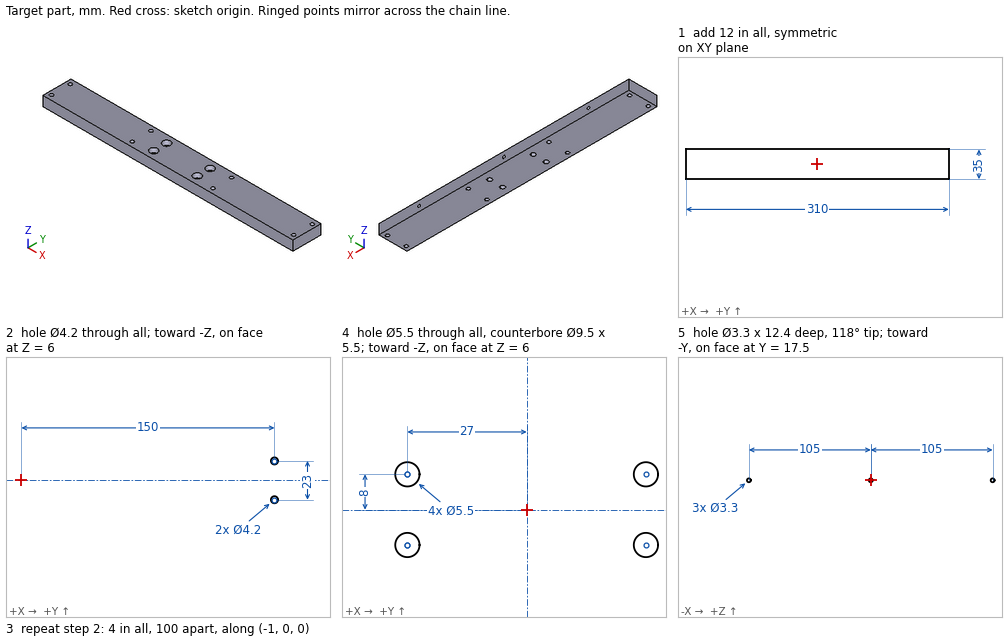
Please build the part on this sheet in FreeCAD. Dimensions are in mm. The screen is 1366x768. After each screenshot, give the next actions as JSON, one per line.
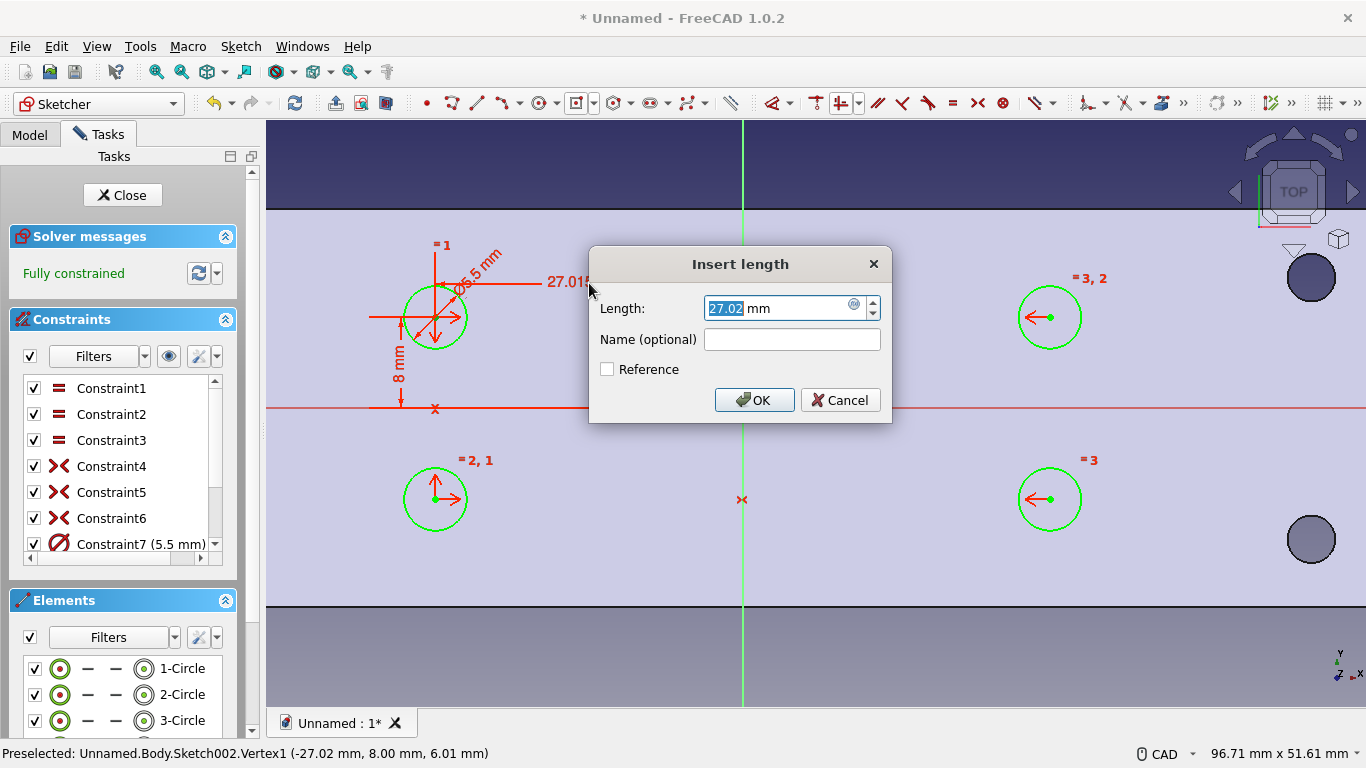
{"action": "type", "text": "27"}
{"action": "key", "text": "Return"}
{"action": "key", "text": "Escape"}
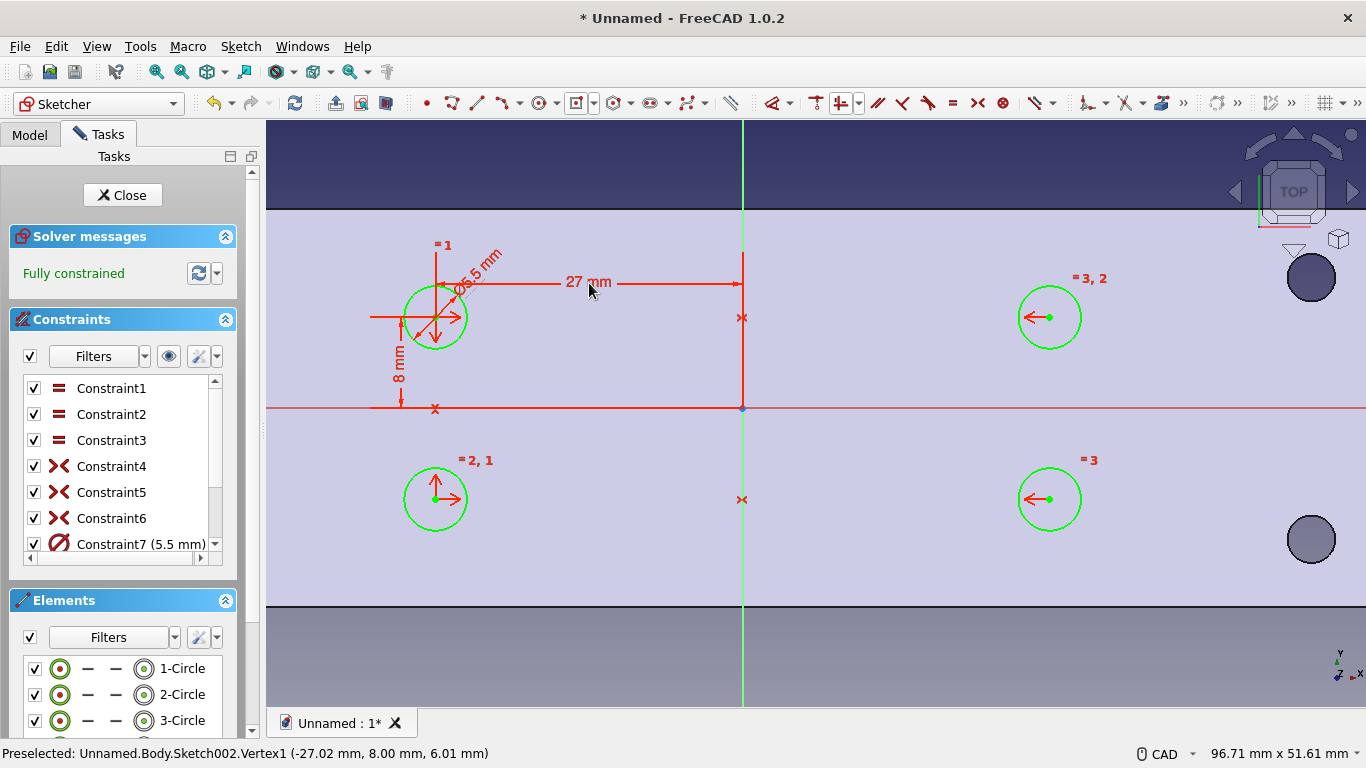
{"action": "left_click", "coordinate": [123, 195]}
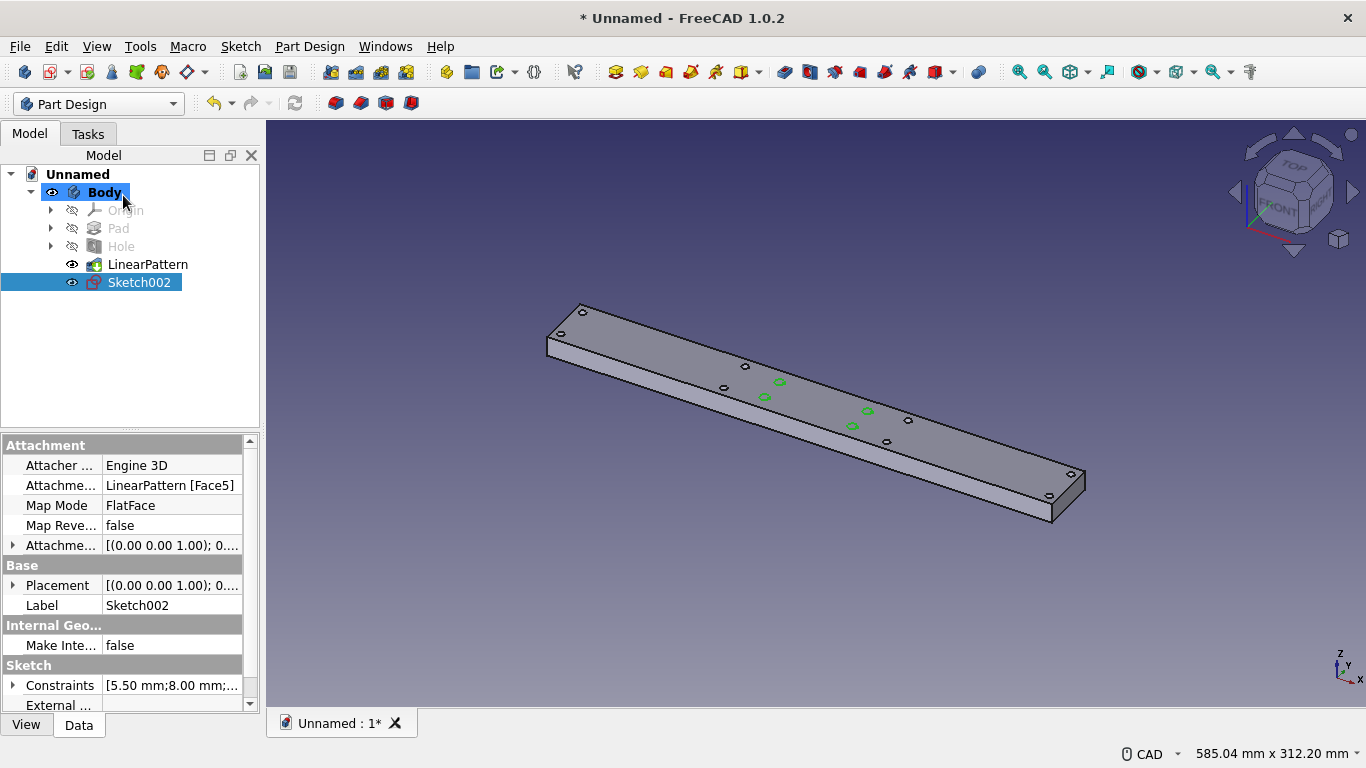
{"action": "left_click", "coordinate": [810, 72]}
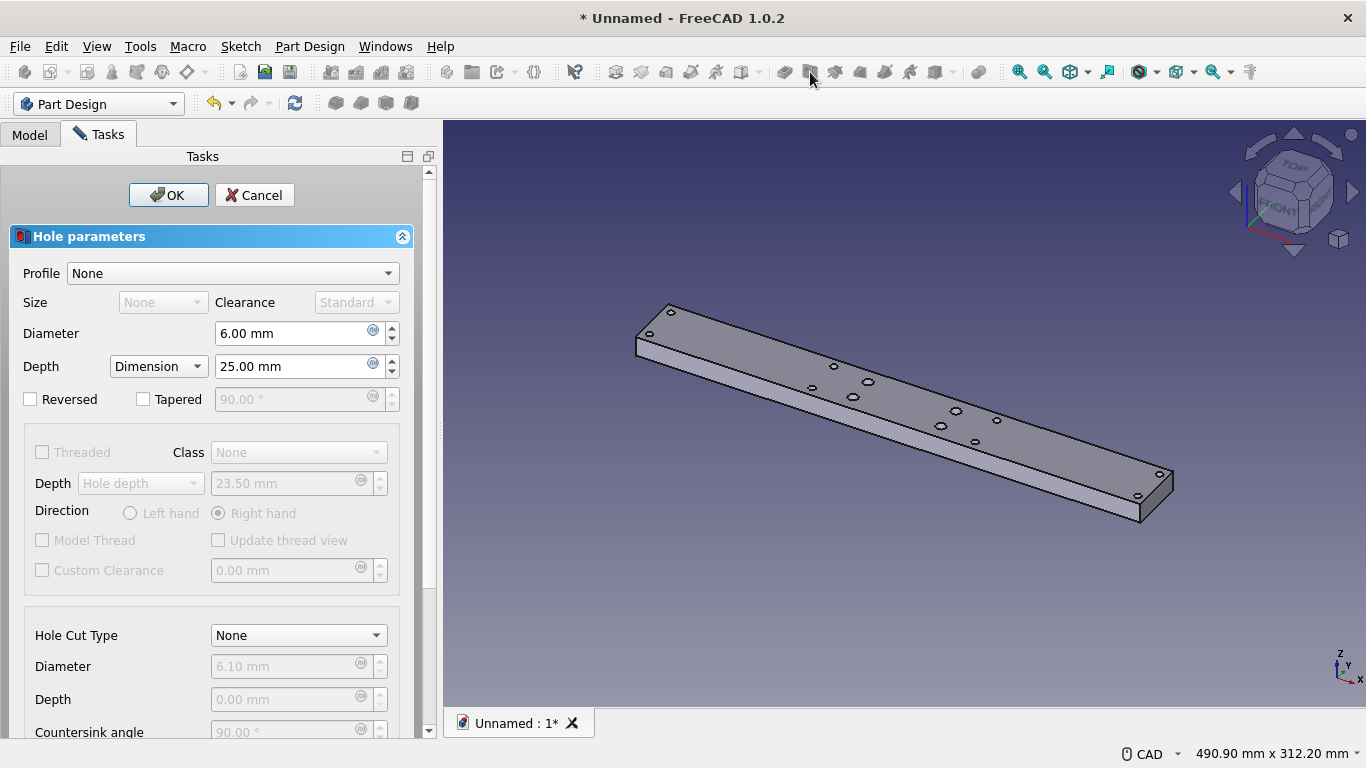
{"action": "triple_click", "coordinate": [300, 334]}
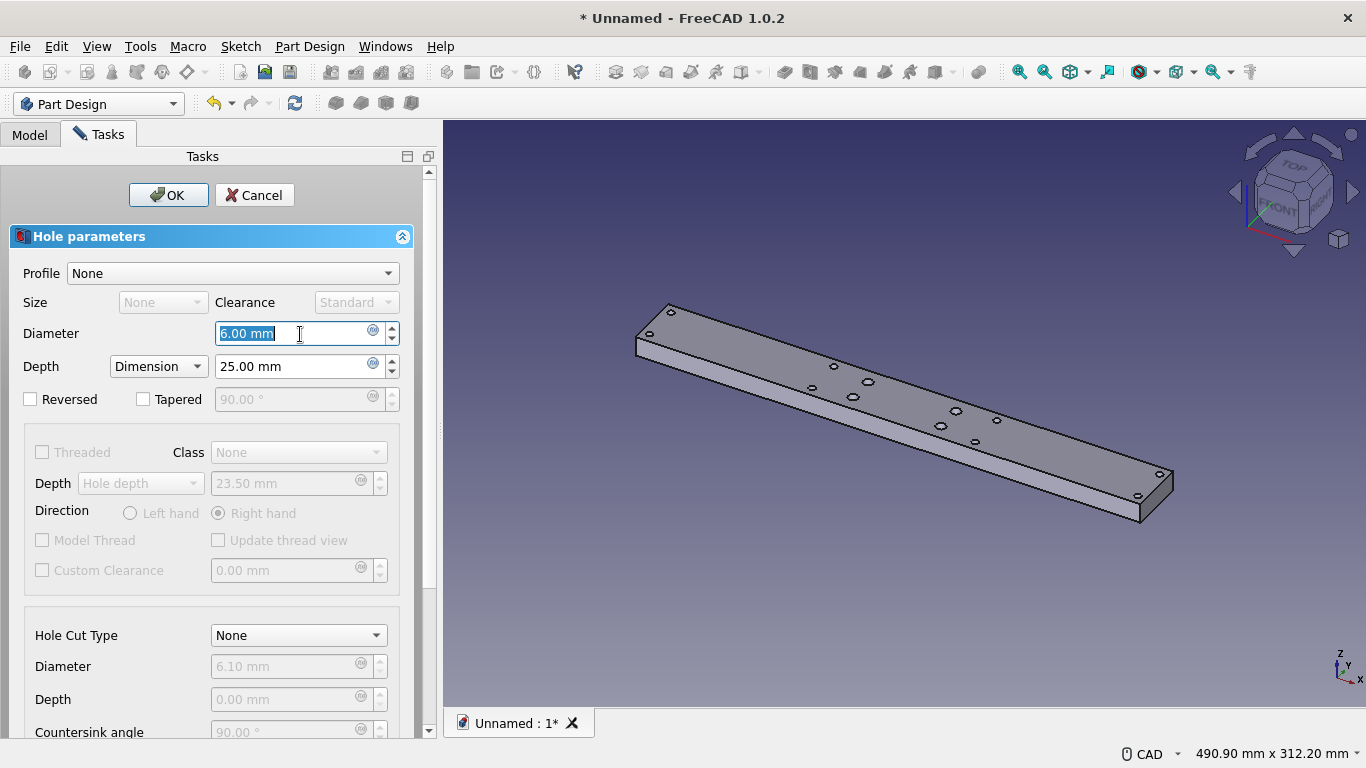
{"action": "type", "text": "5.5"}
{"action": "key", "text": "Tab"}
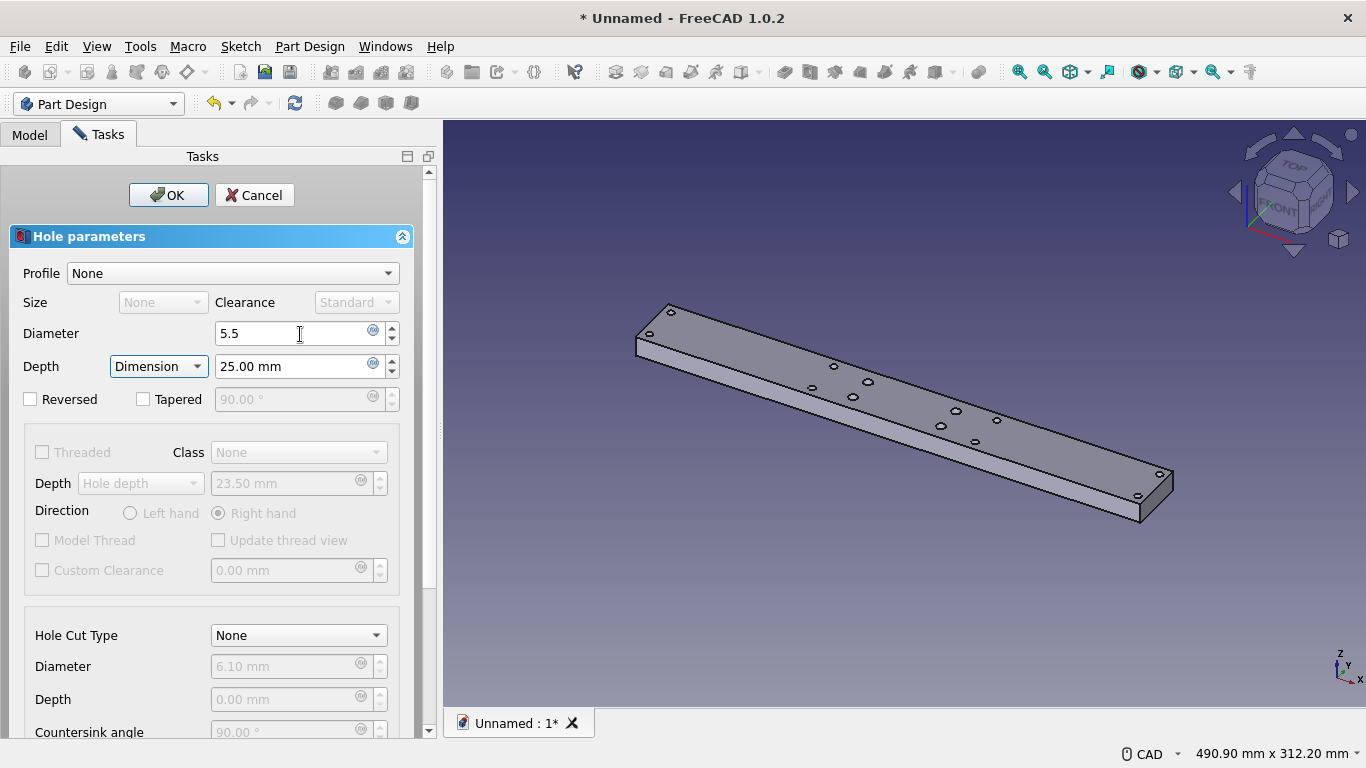
{"action": "left_click", "coordinate": [160, 366]}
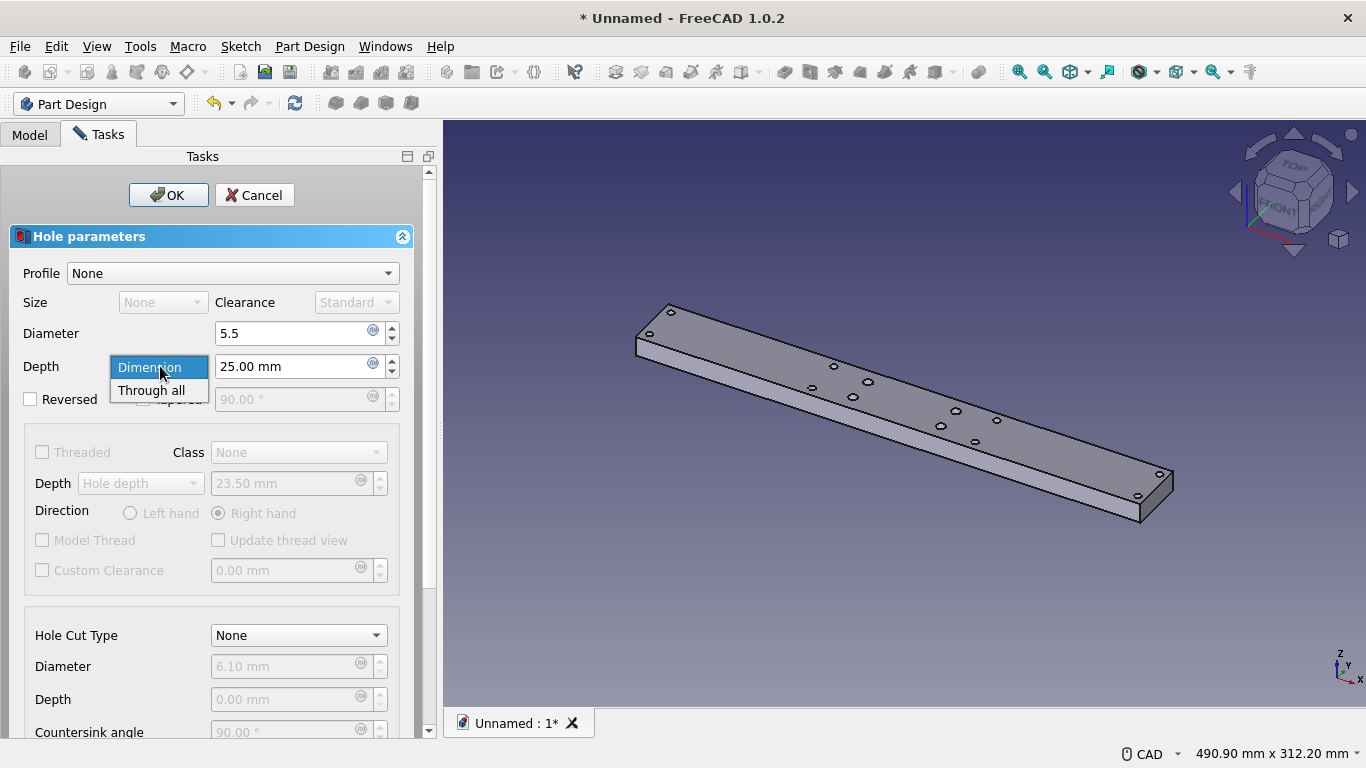
{"action": "left_click", "coordinate": [158, 390]}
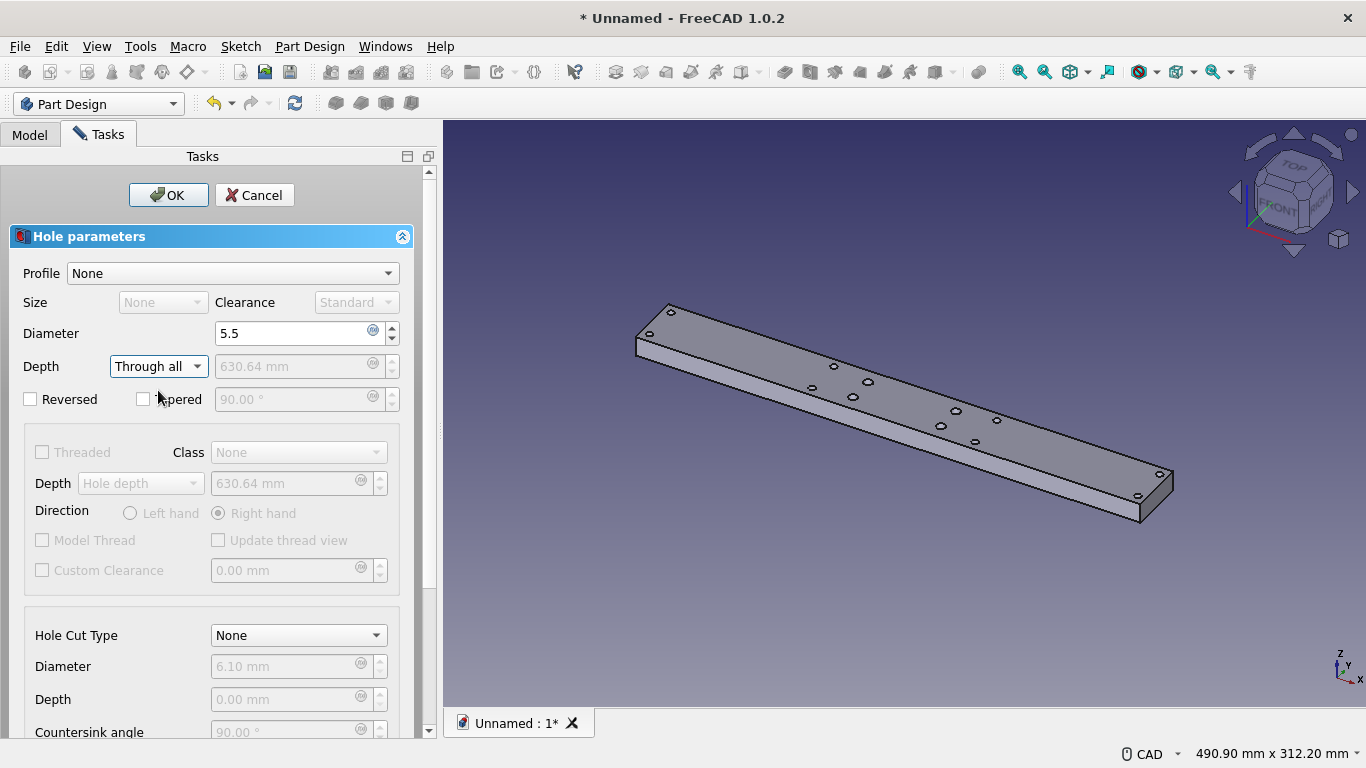
{"action": "left_click", "coordinate": [300, 636]}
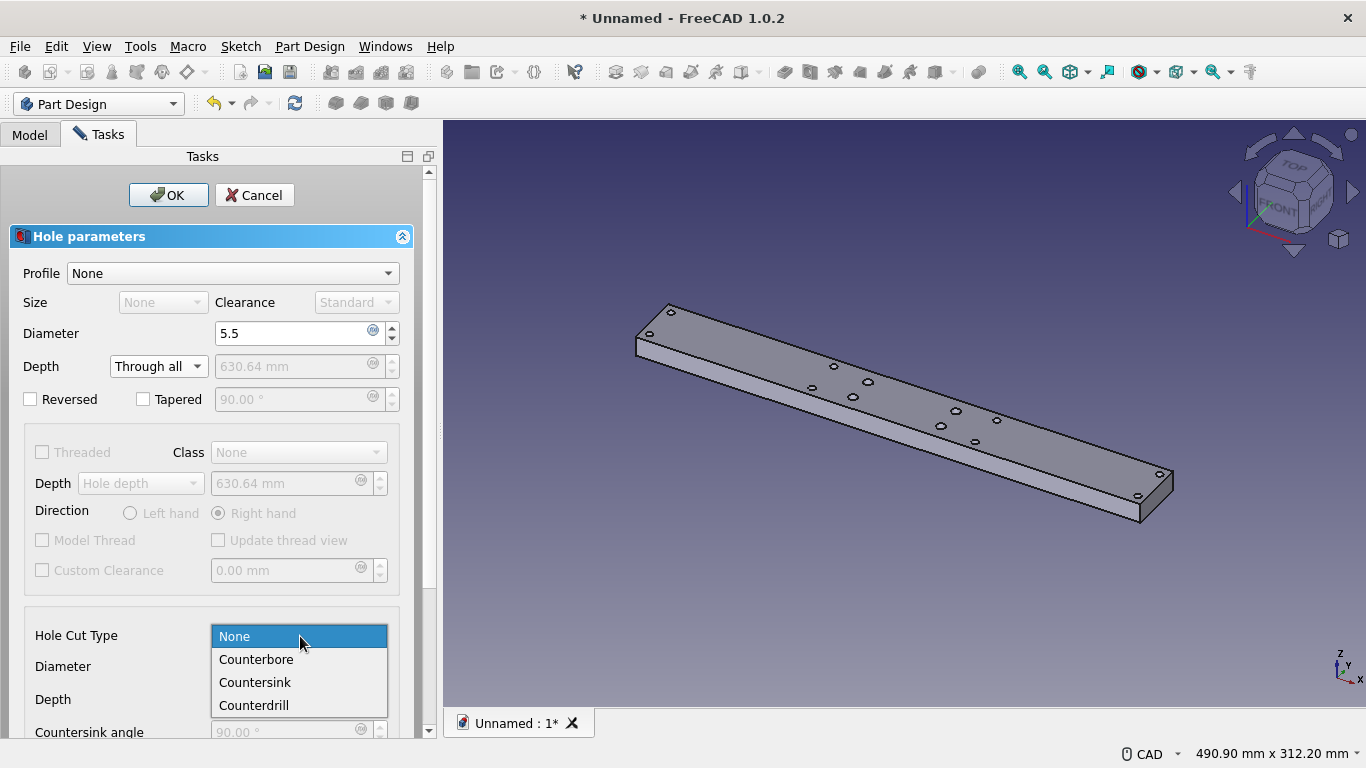
{"action": "left_click", "coordinate": [298, 660]}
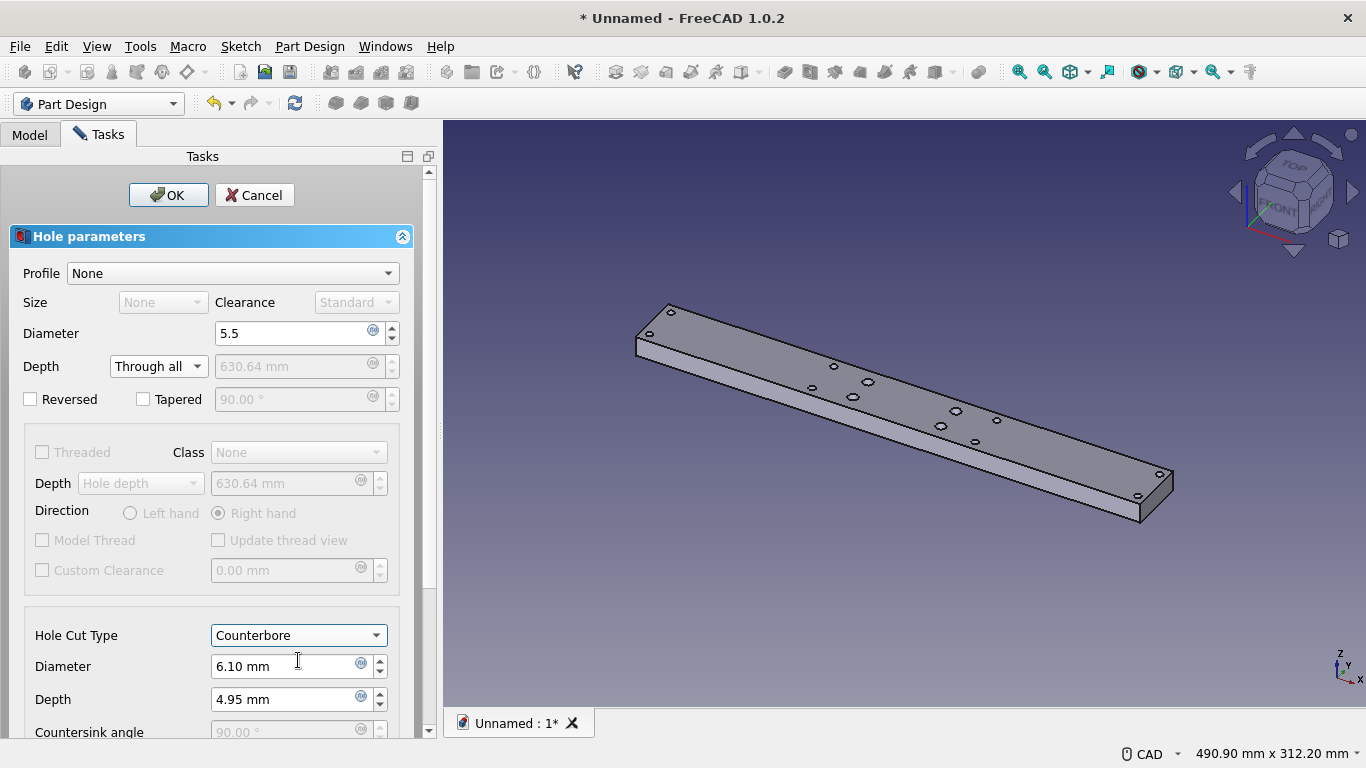
{"action": "triple_click", "coordinate": [292, 666]}